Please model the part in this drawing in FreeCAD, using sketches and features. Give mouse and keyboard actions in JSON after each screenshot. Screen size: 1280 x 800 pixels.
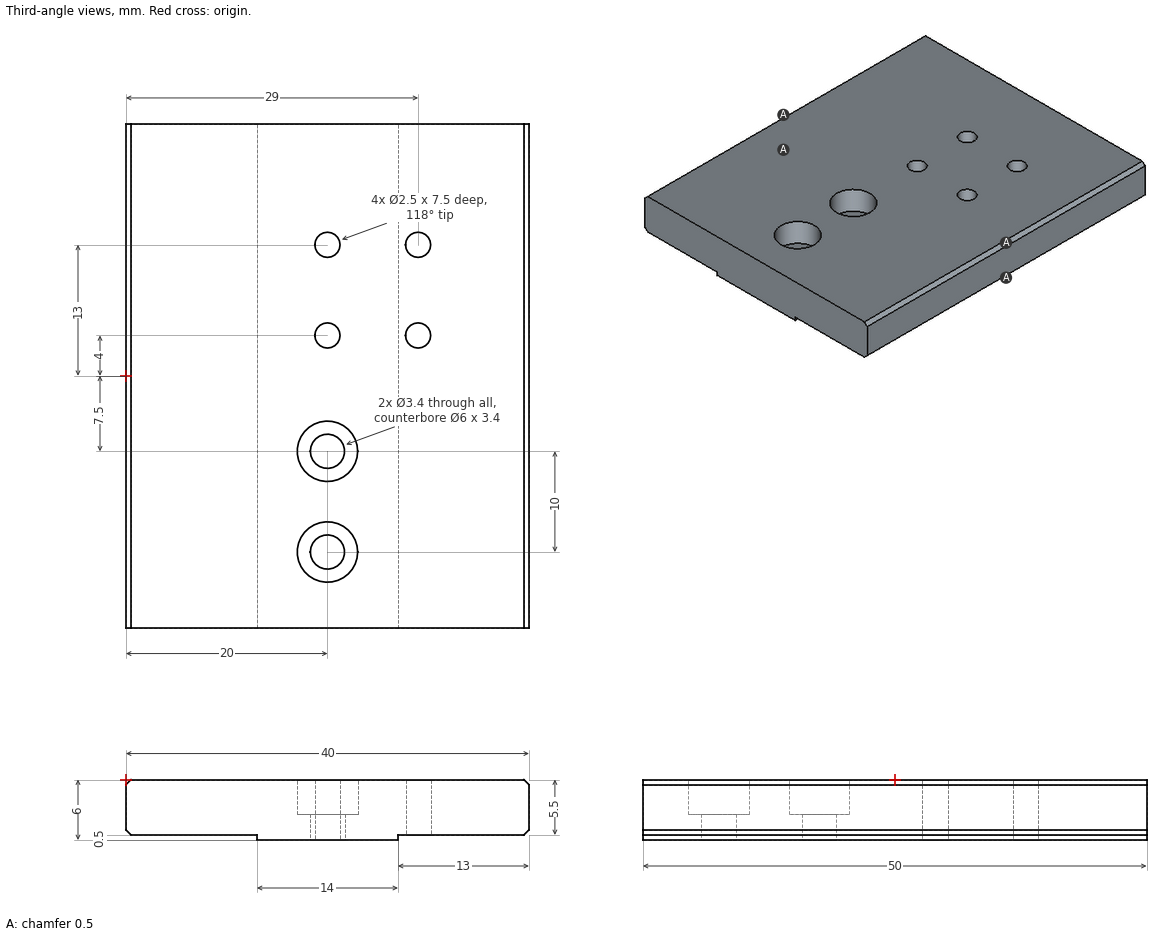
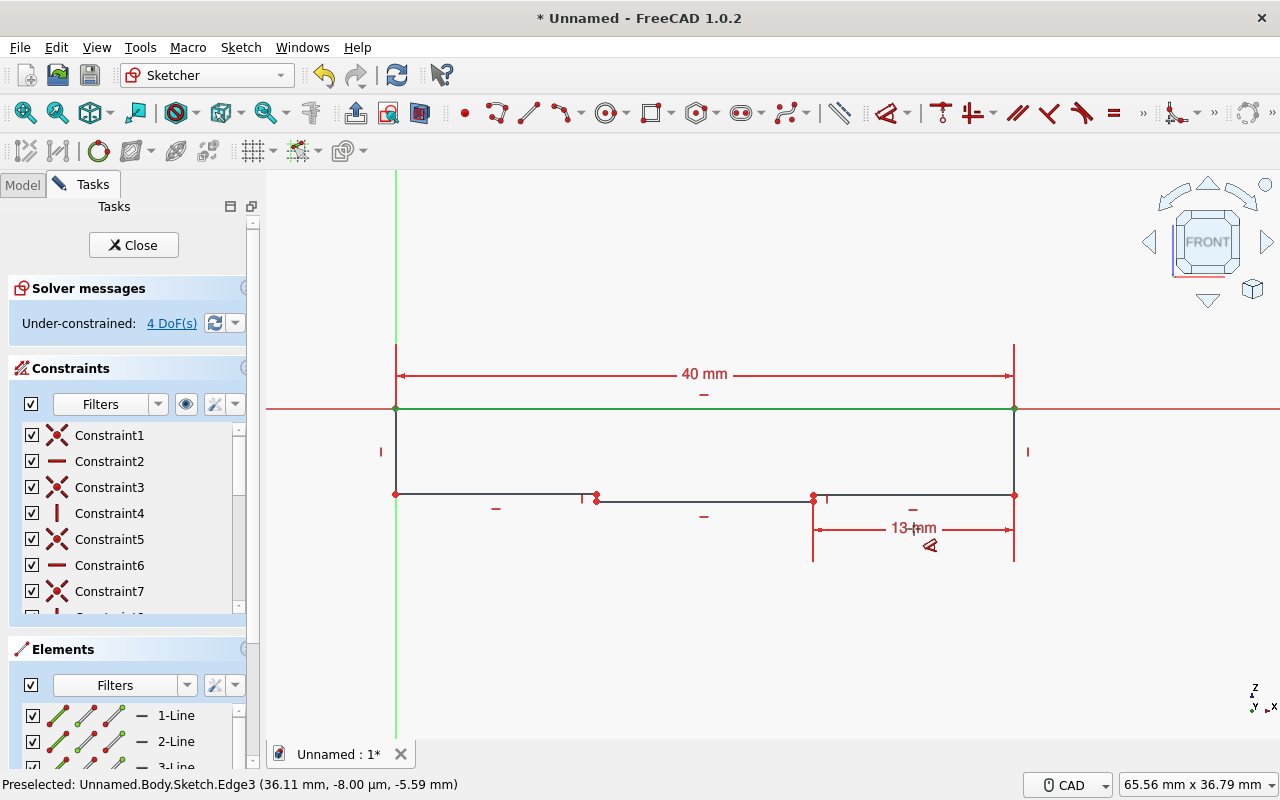
{"action": "left_click", "coordinate": [748, 502]}
{"action": "left_click", "coordinate": [705, 536]}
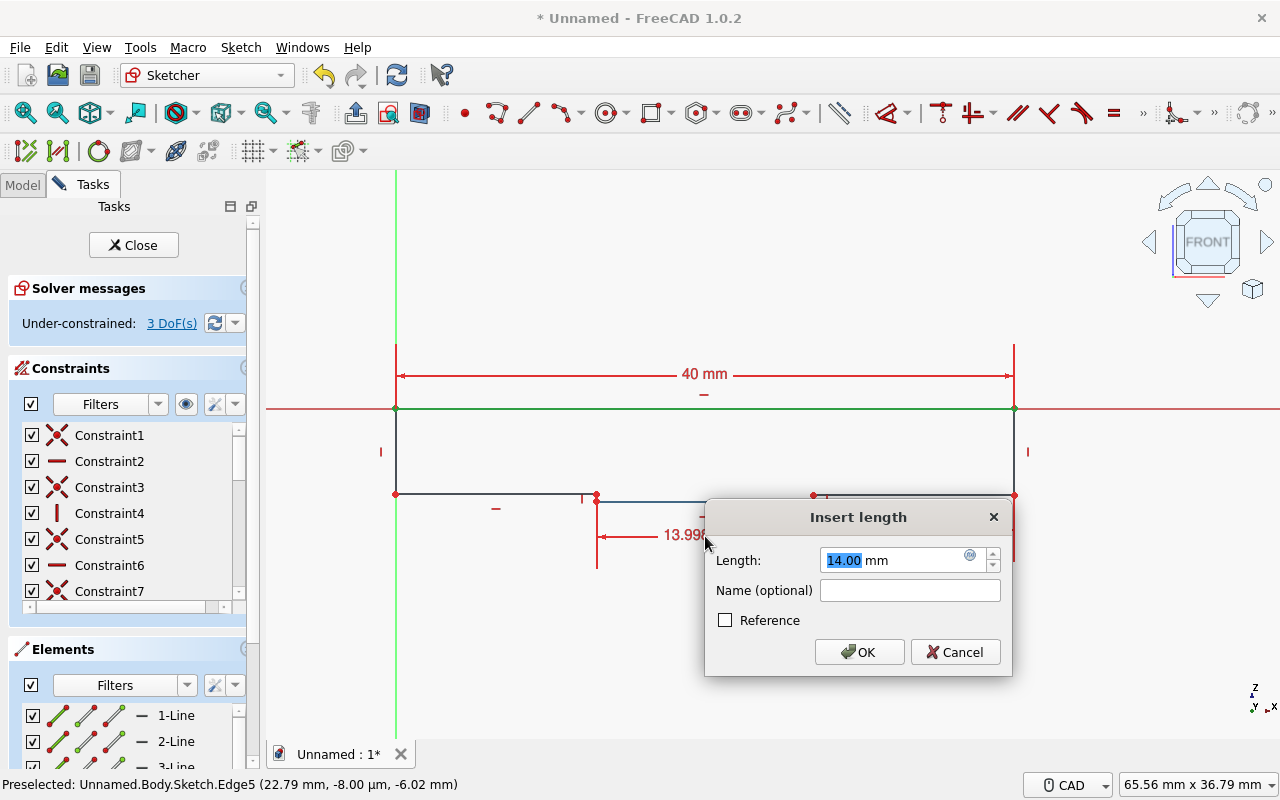
{"action": "type", "text": "14"}
{"action": "key", "text": "Return"}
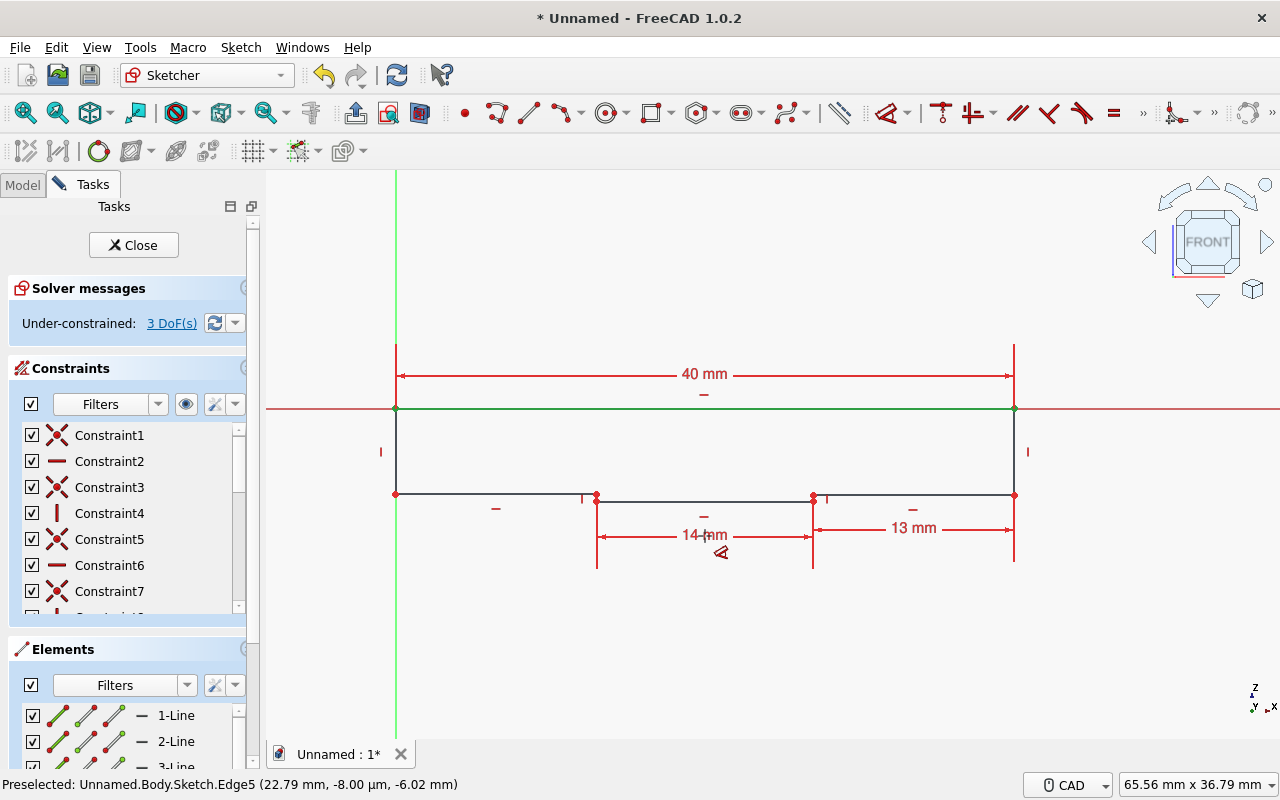
{"action": "scroll", "coordinate": [813, 502], "scroll_direction": "up", "scroll_amount": 3}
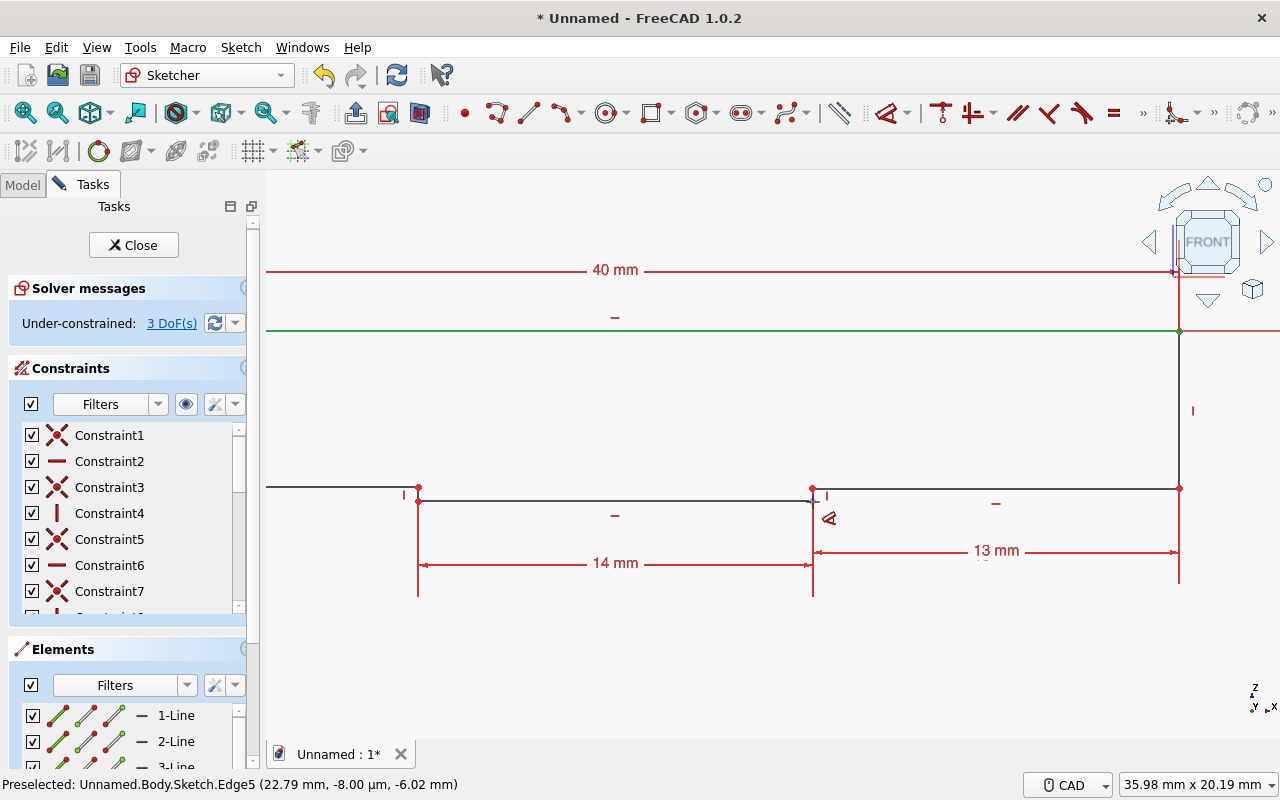
{"action": "left_click", "coordinate": [813, 501]}
{"action": "left_click", "coordinate": [847, 416]}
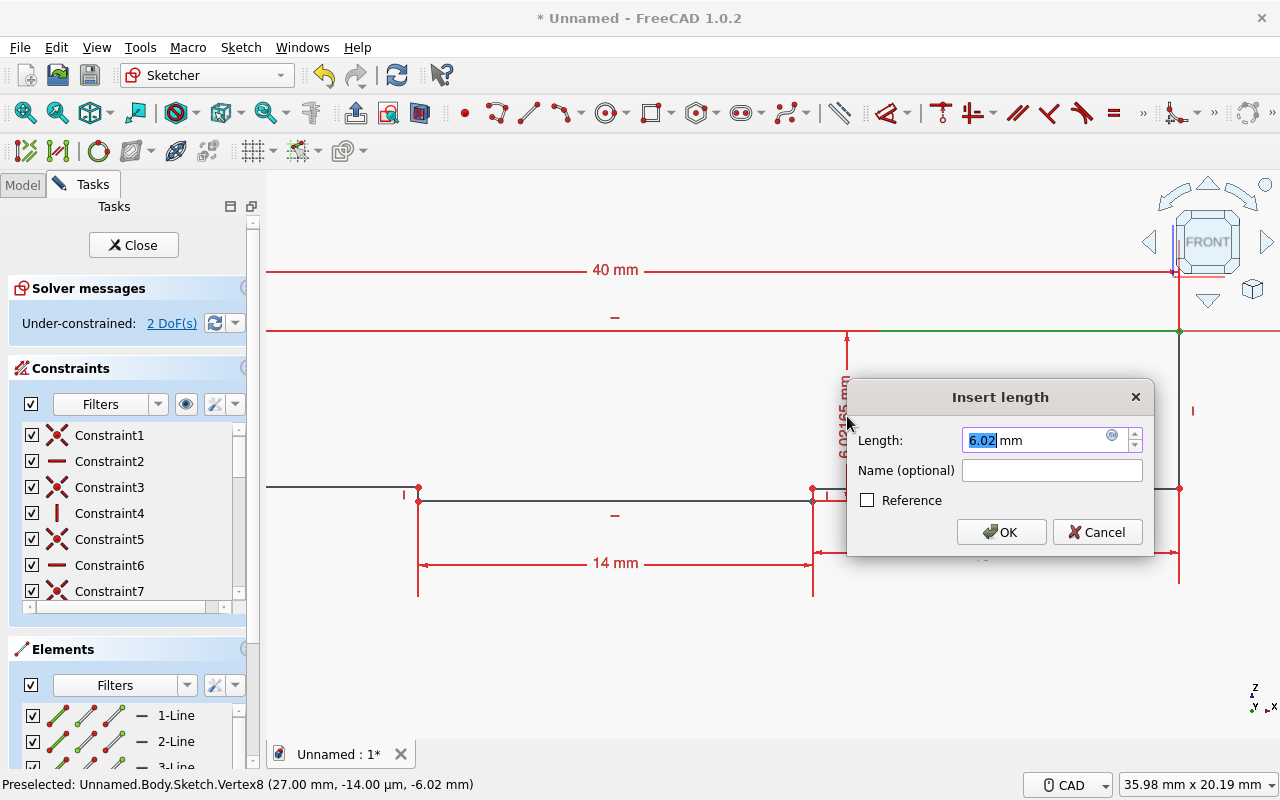
{"action": "type", "text": "6"}
{"action": "key", "text": "Return"}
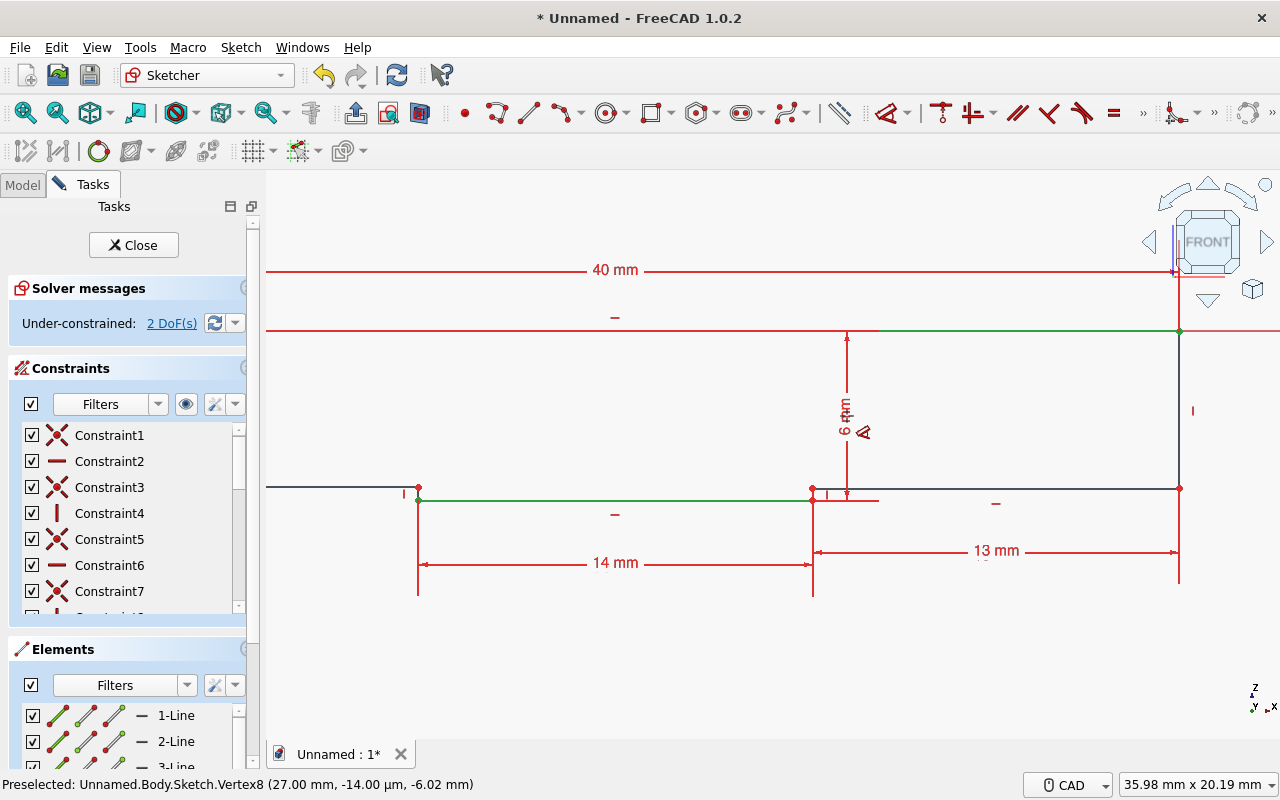
{"action": "scroll", "coordinate": [813, 501], "scroll_direction": "down", "scroll_amount": 3}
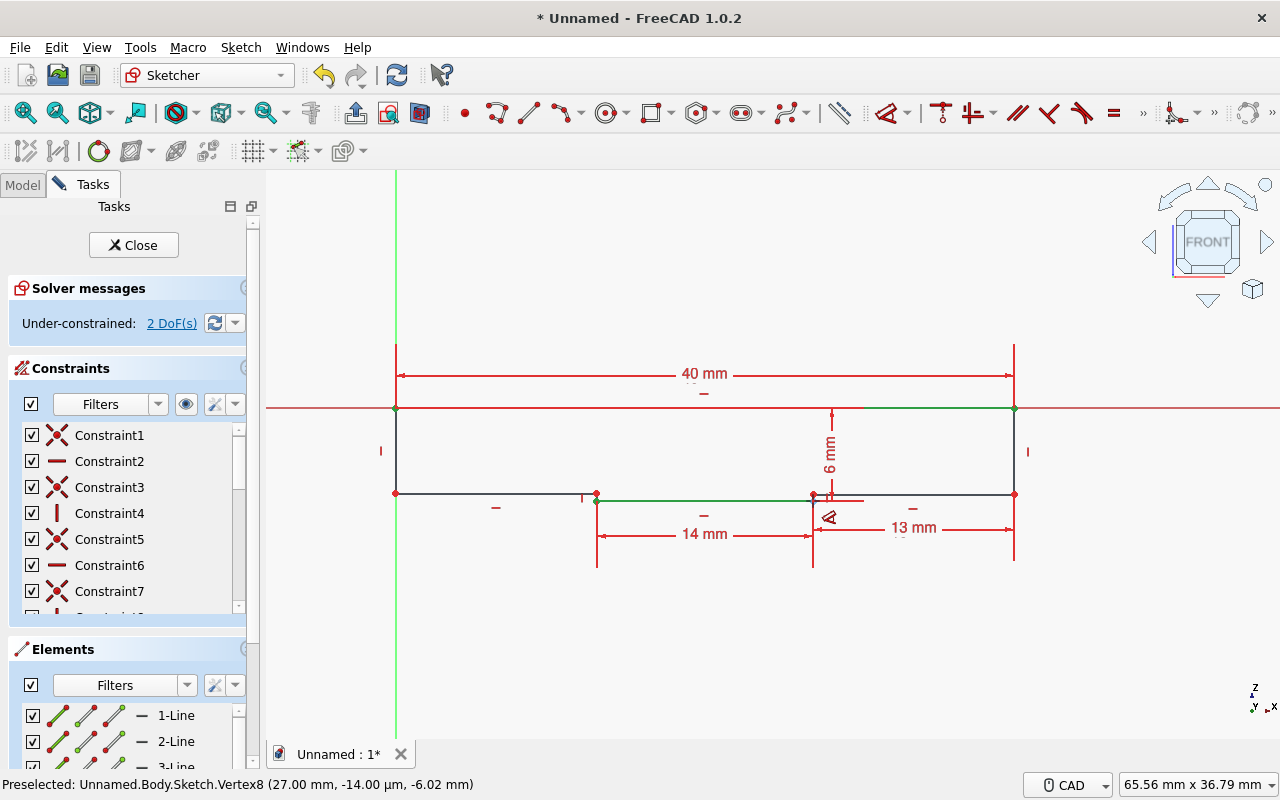
{"action": "left_click", "coordinate": [1014, 434]}
{"action": "left_click", "coordinate": [1048, 451]}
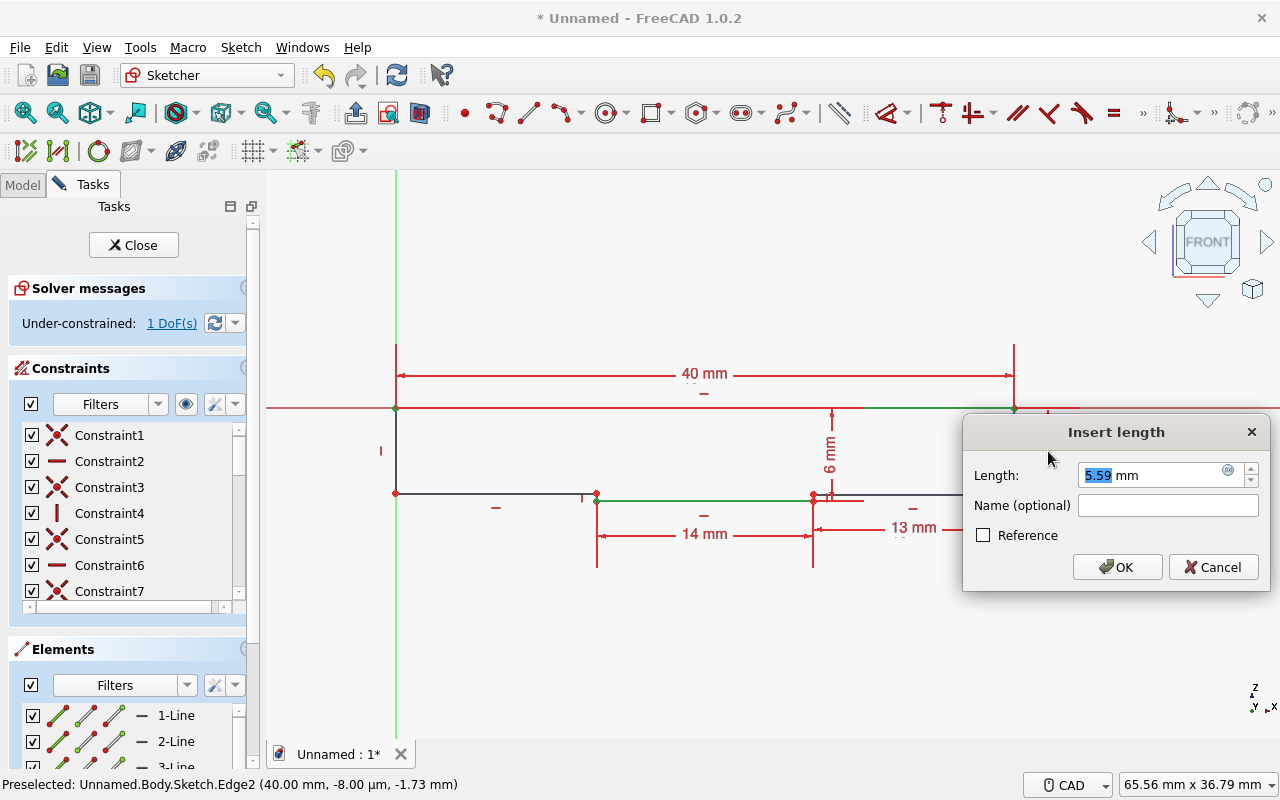
{"action": "type", "text": "5.5"}
{"action": "key", "text": "Return"}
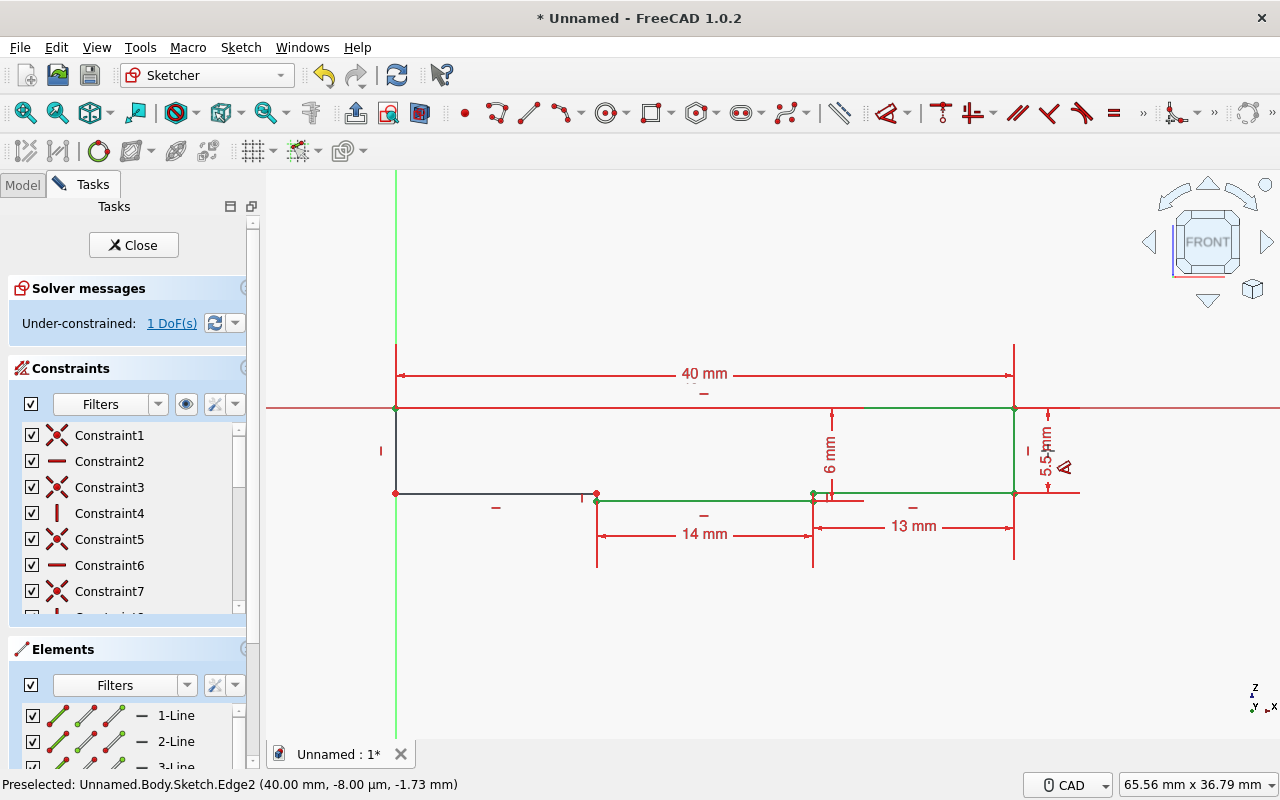
{"action": "scroll", "coordinate": [597, 497], "scroll_direction": "up", "scroll_amount": 9}